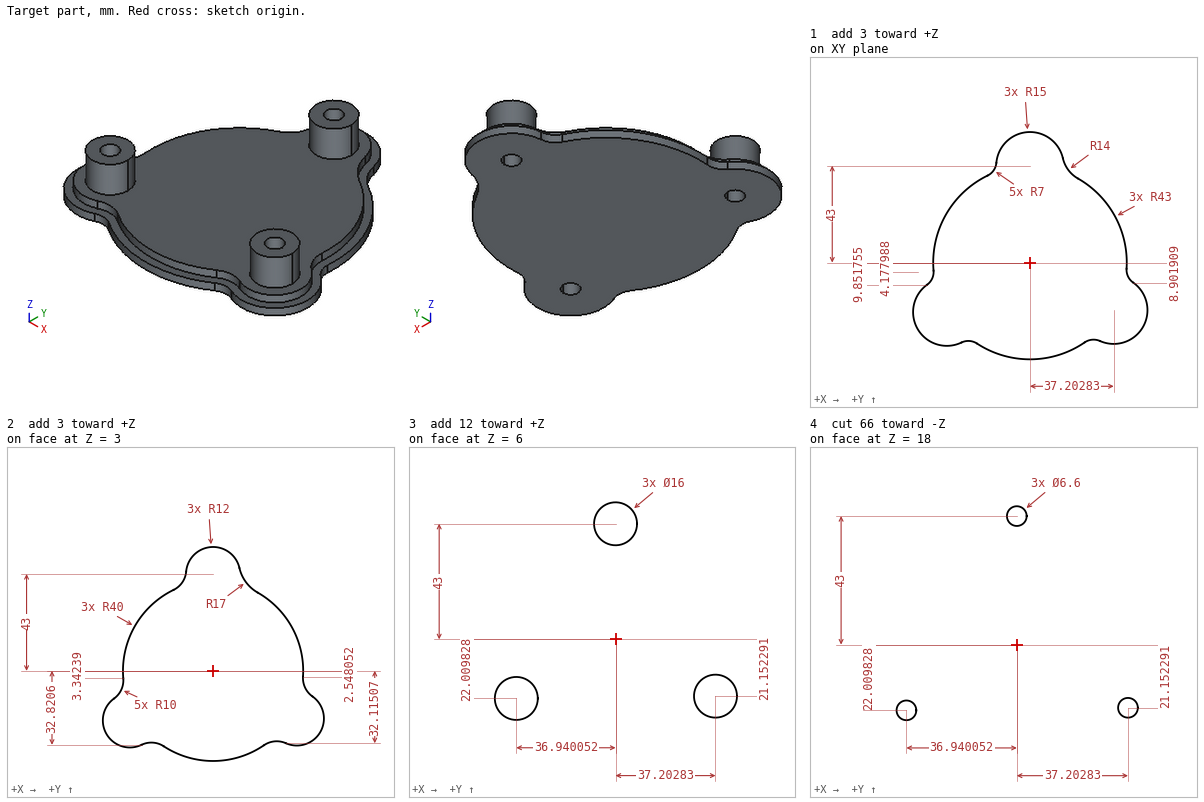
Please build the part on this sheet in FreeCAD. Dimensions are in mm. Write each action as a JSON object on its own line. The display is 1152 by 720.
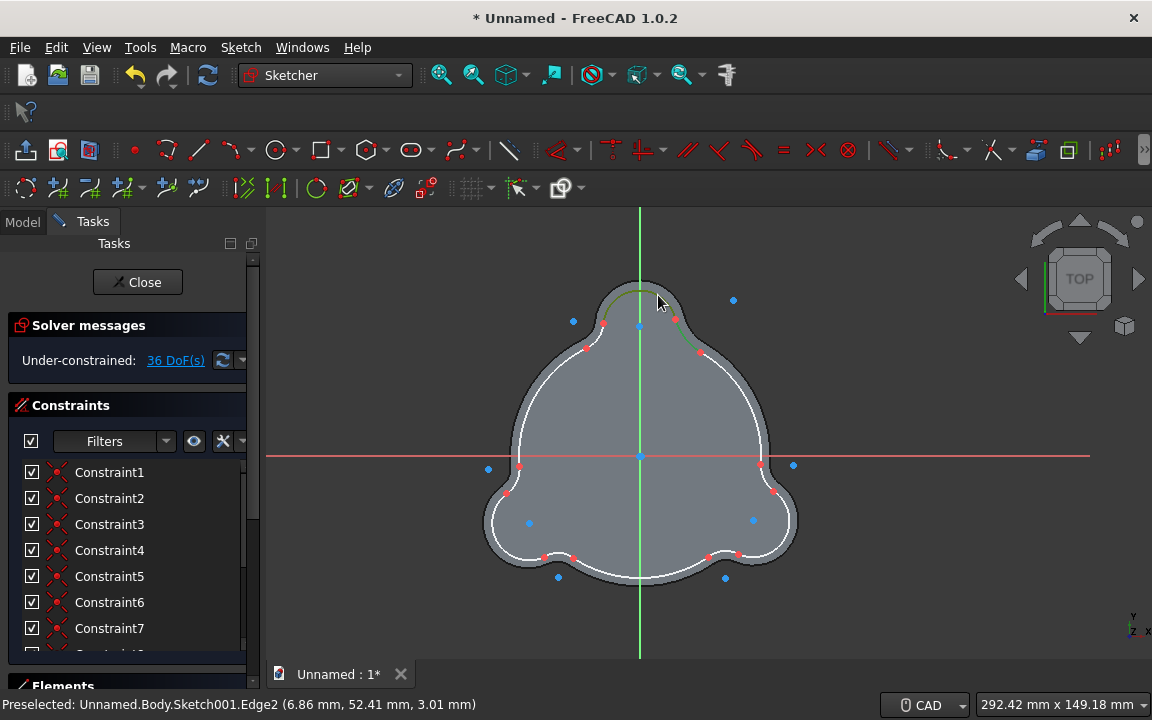
{"action": "left_click", "coordinate": [752, 150]}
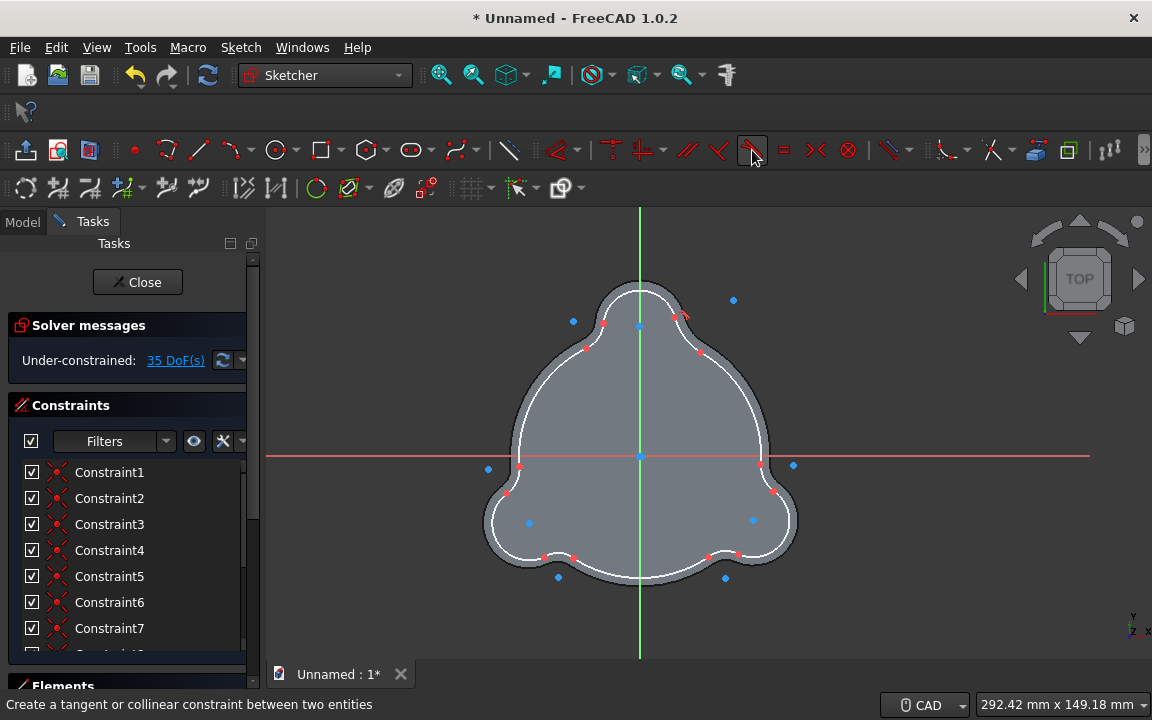
{"action": "left_click", "coordinate": [680, 330]}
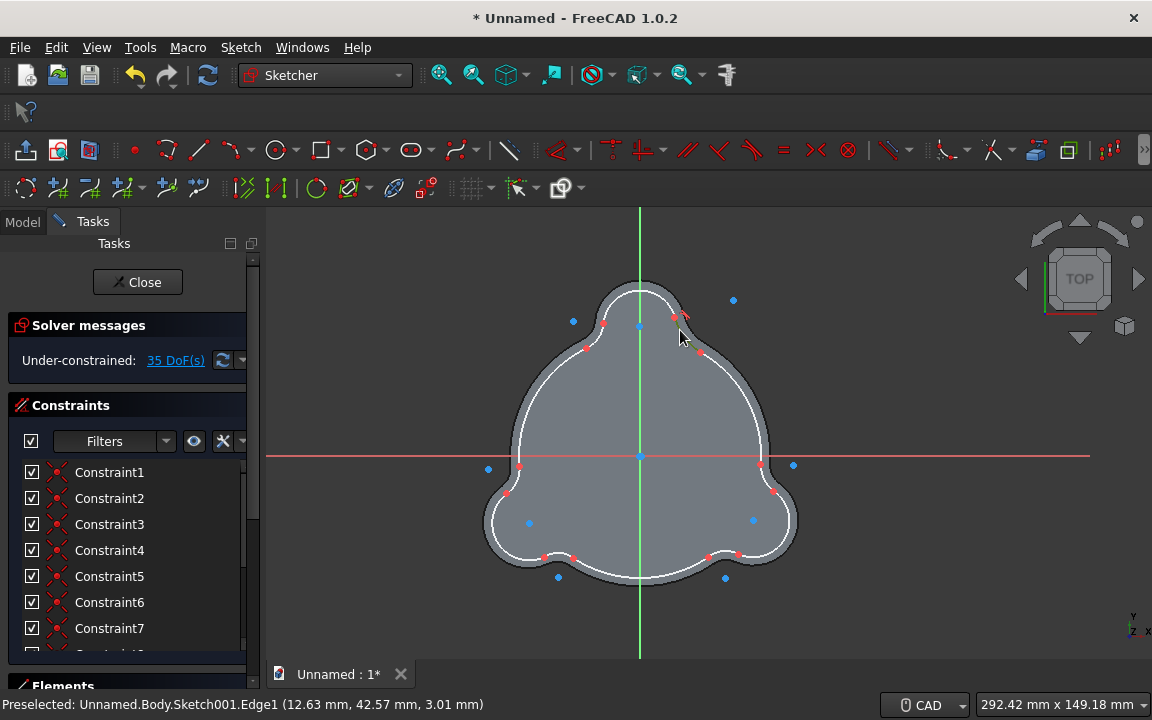
{"action": "left_click", "coordinate": [757, 424]}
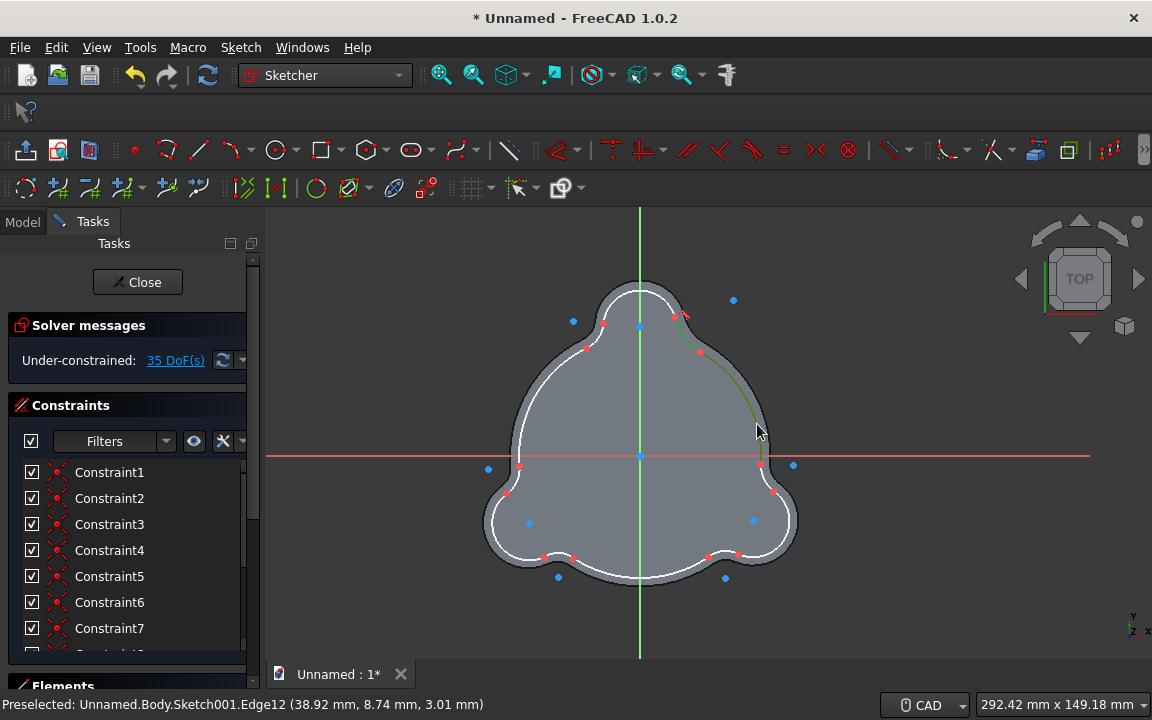
{"action": "key", "text": "t"}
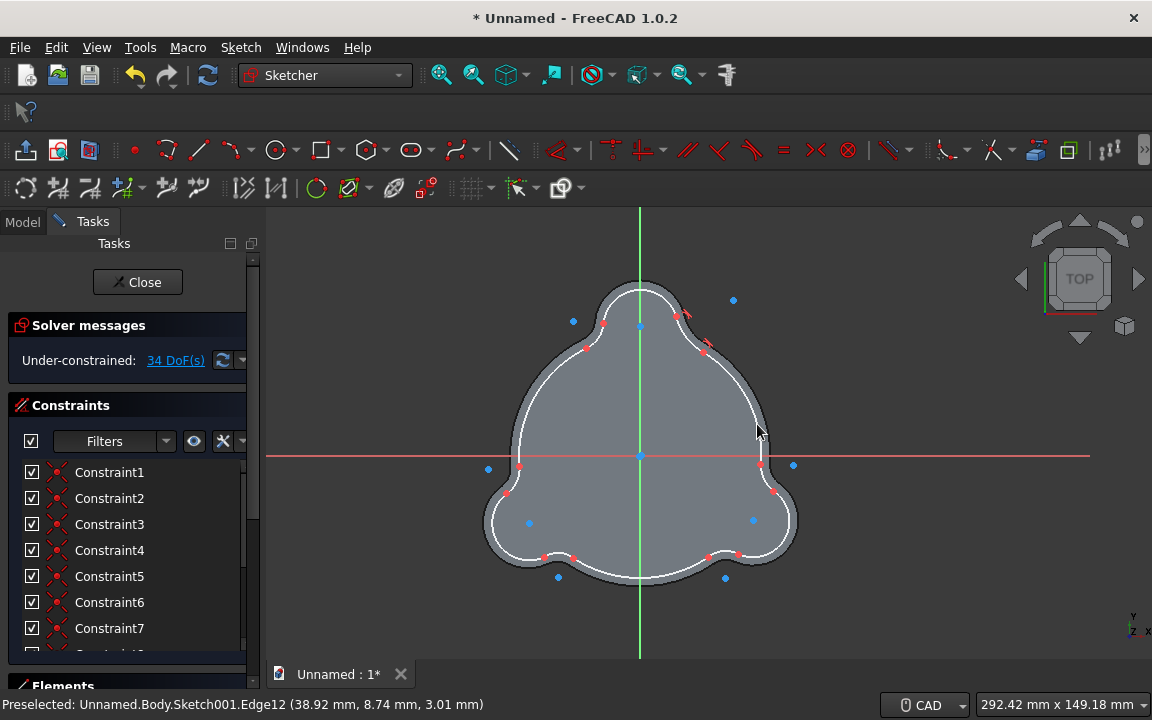
{"action": "left_click", "coordinate": [657, 294]}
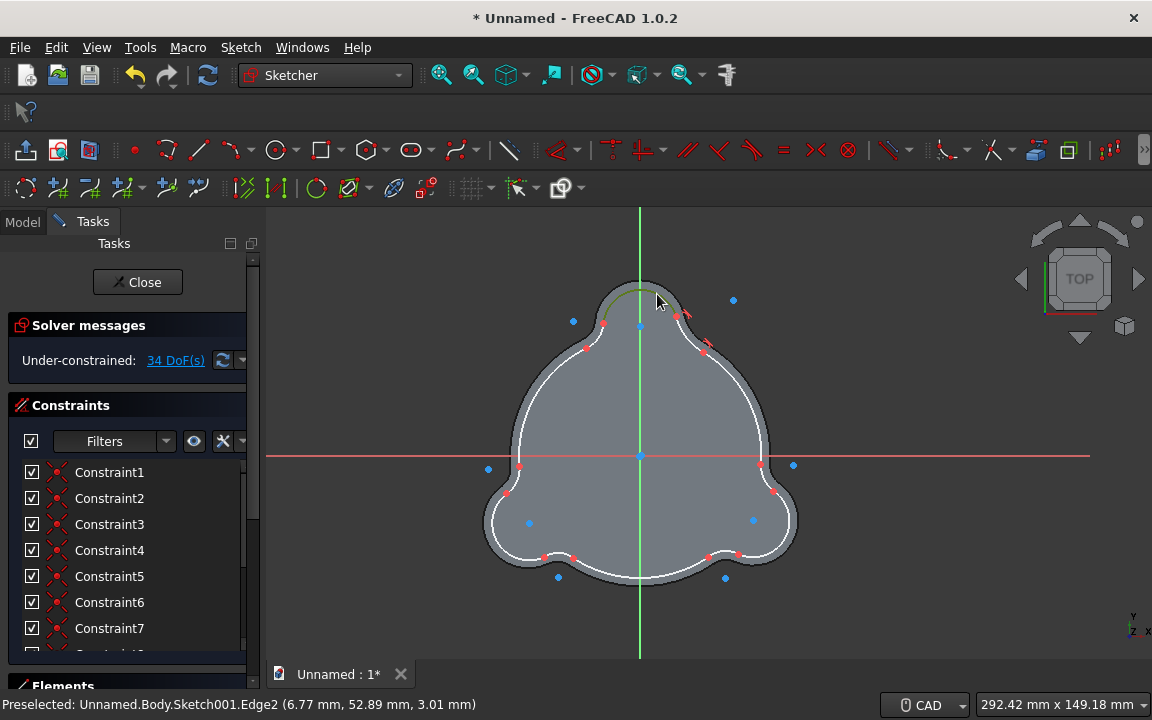
{"action": "scroll", "coordinate": [594, 343], "scroll_direction": "up", "scroll_amount": 2}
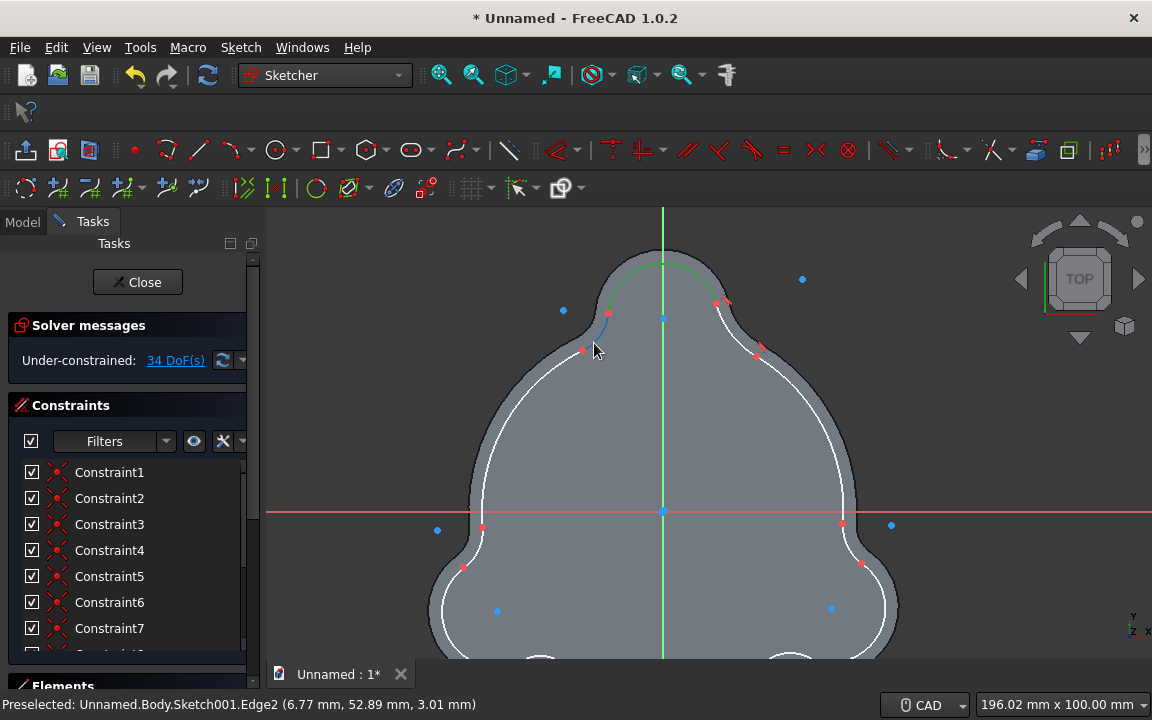
{"action": "left_click", "coordinate": [594, 343]}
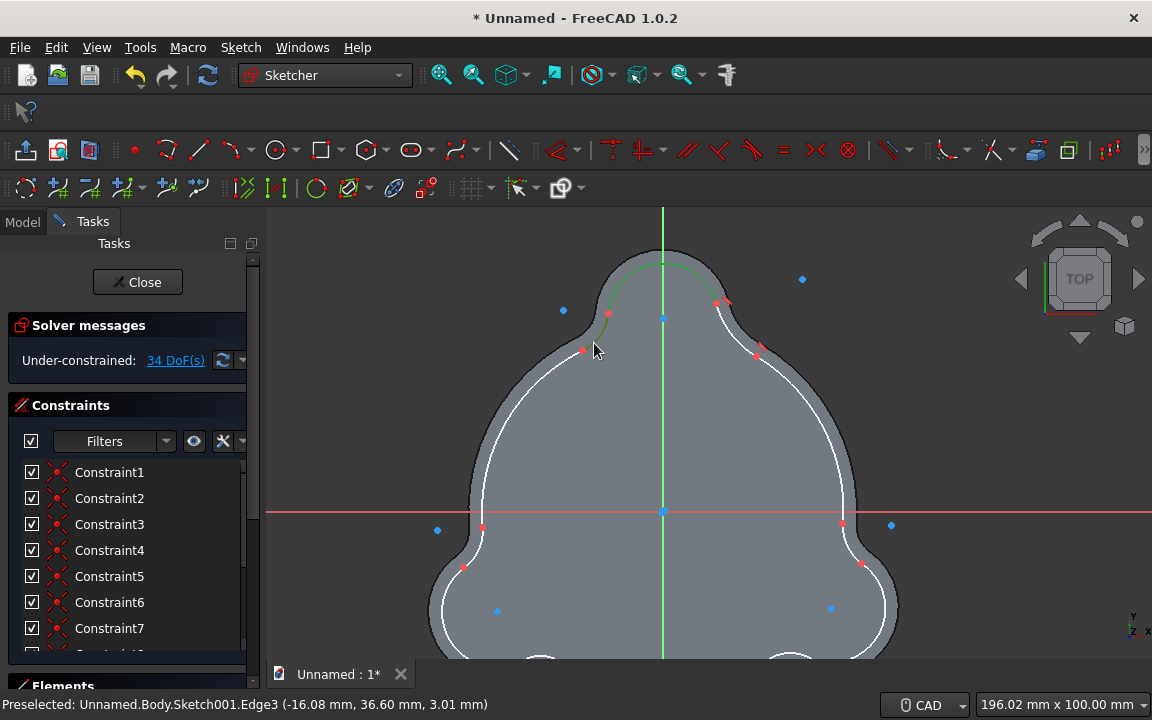
{"action": "left_click", "coordinate": [752, 150]}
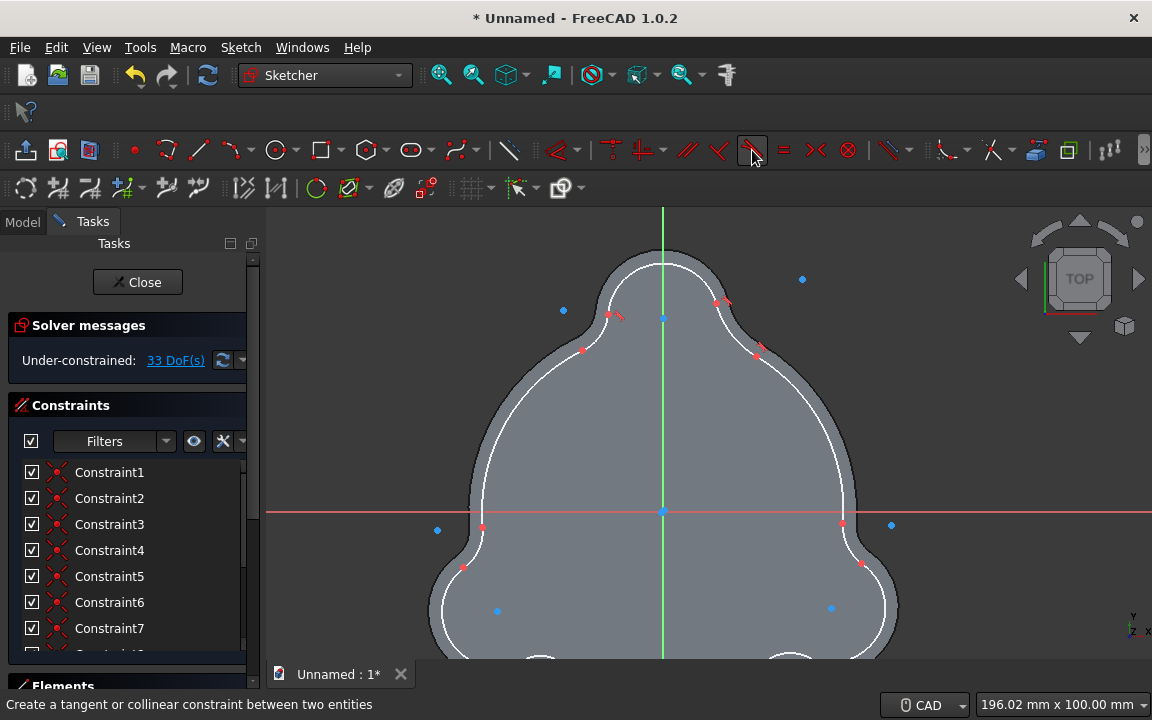
{"action": "left_click", "coordinate": [594, 343]}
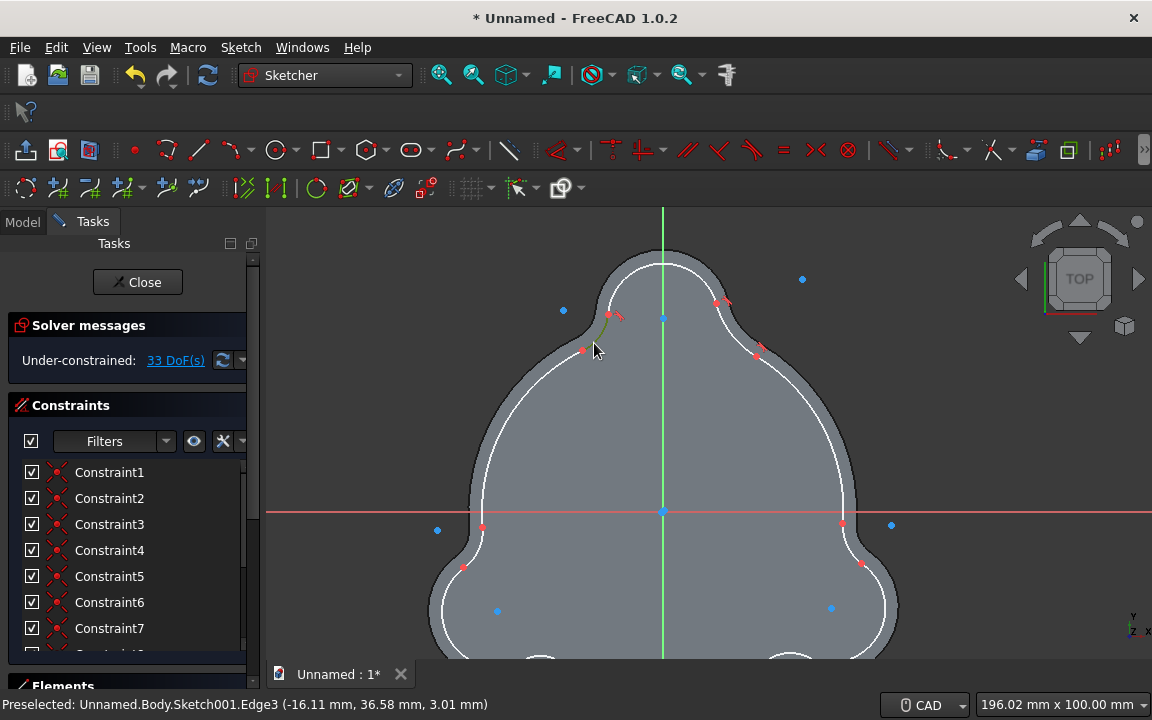
{"action": "left_click", "coordinate": [531, 389]}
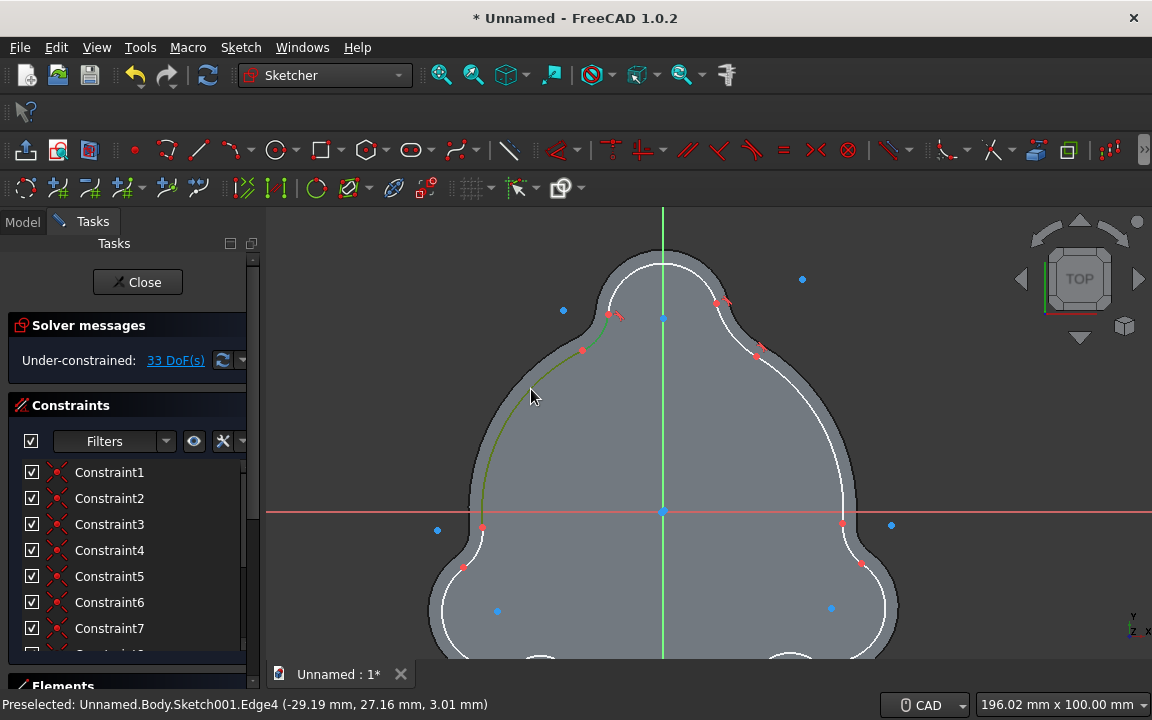
{"action": "left_click", "coordinate": [752, 150]}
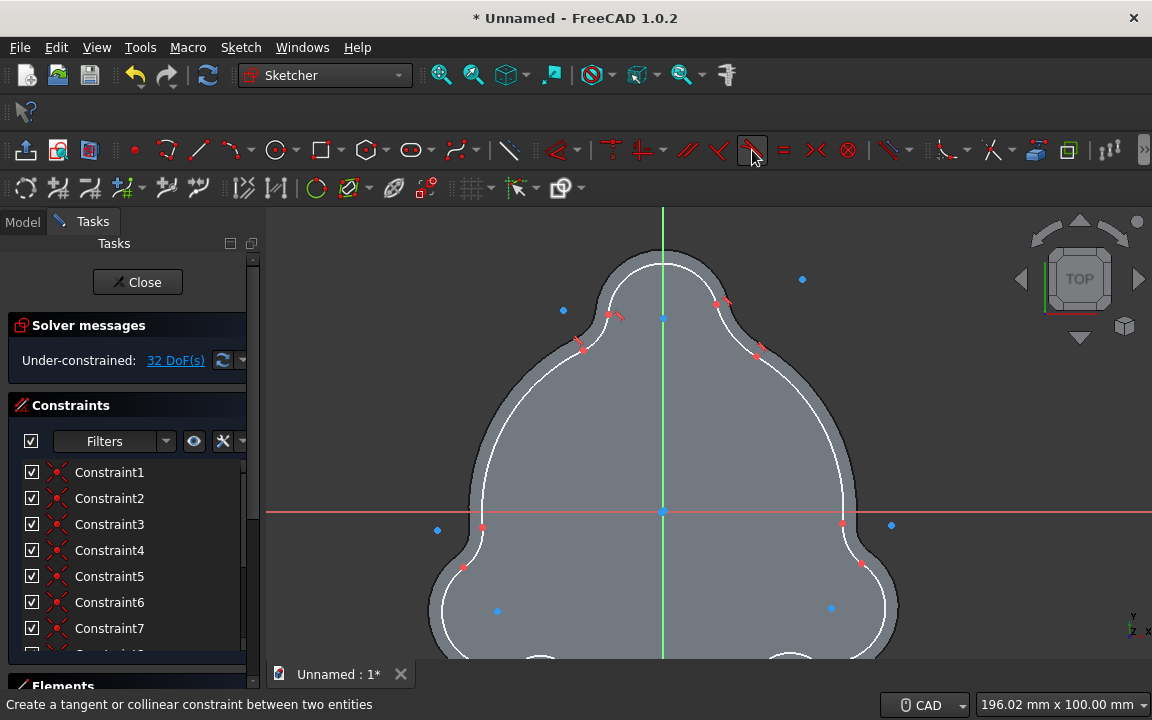
{"action": "left_click", "coordinate": [531, 389]}